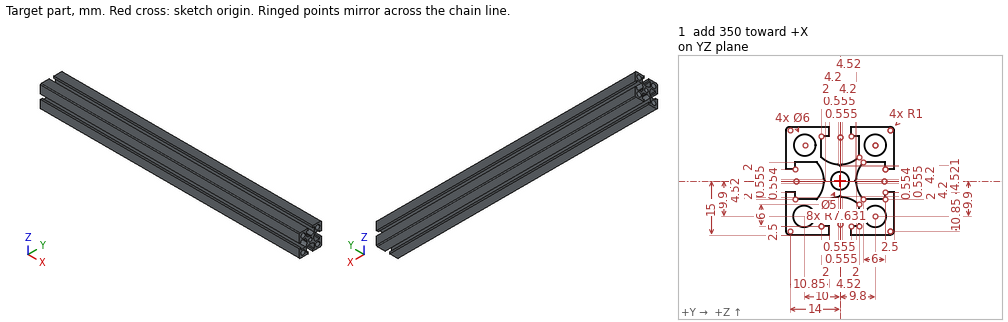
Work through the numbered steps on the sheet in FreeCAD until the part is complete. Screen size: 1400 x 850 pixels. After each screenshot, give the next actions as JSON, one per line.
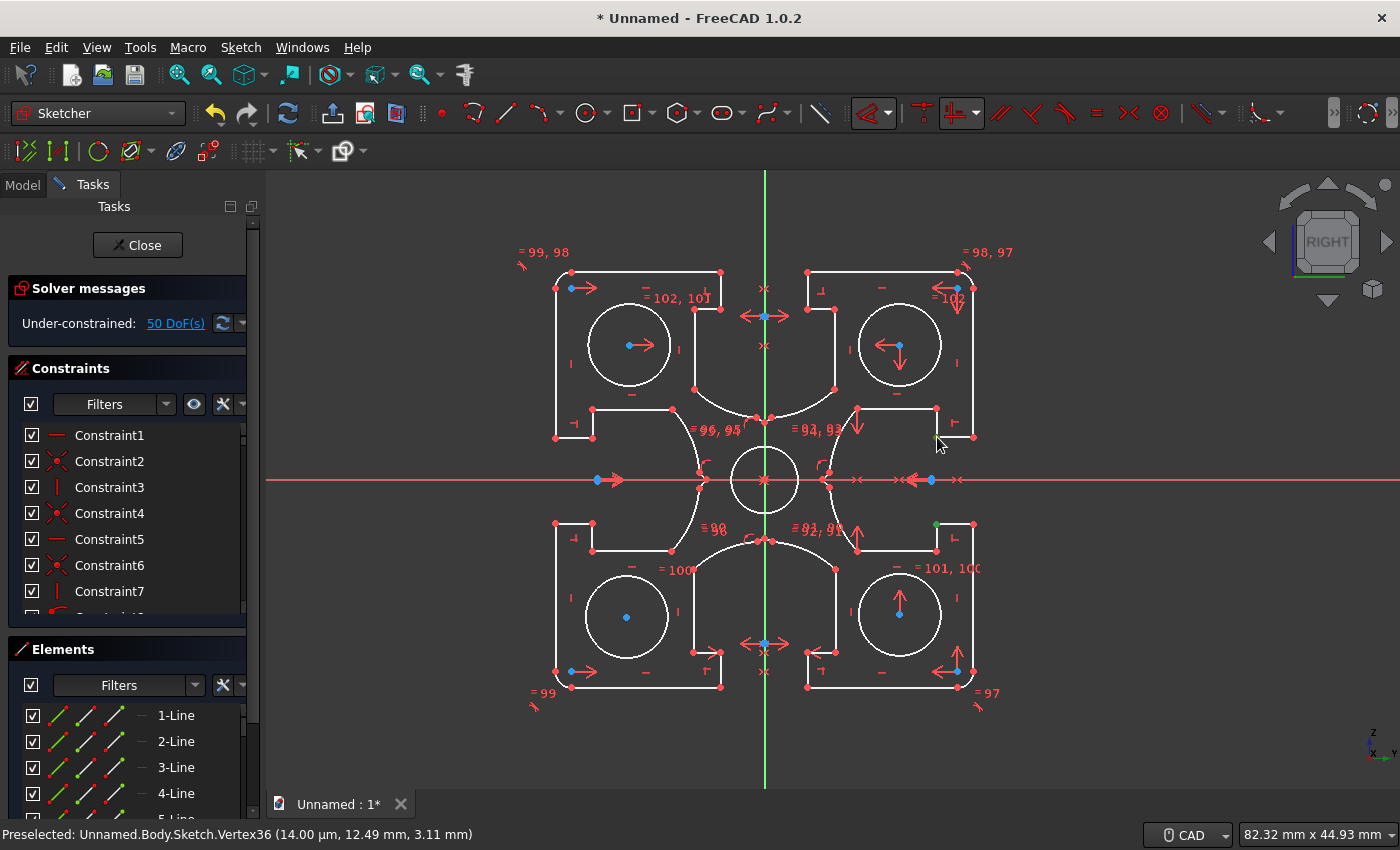
{"action": "left_click", "coordinate": [361, 480]}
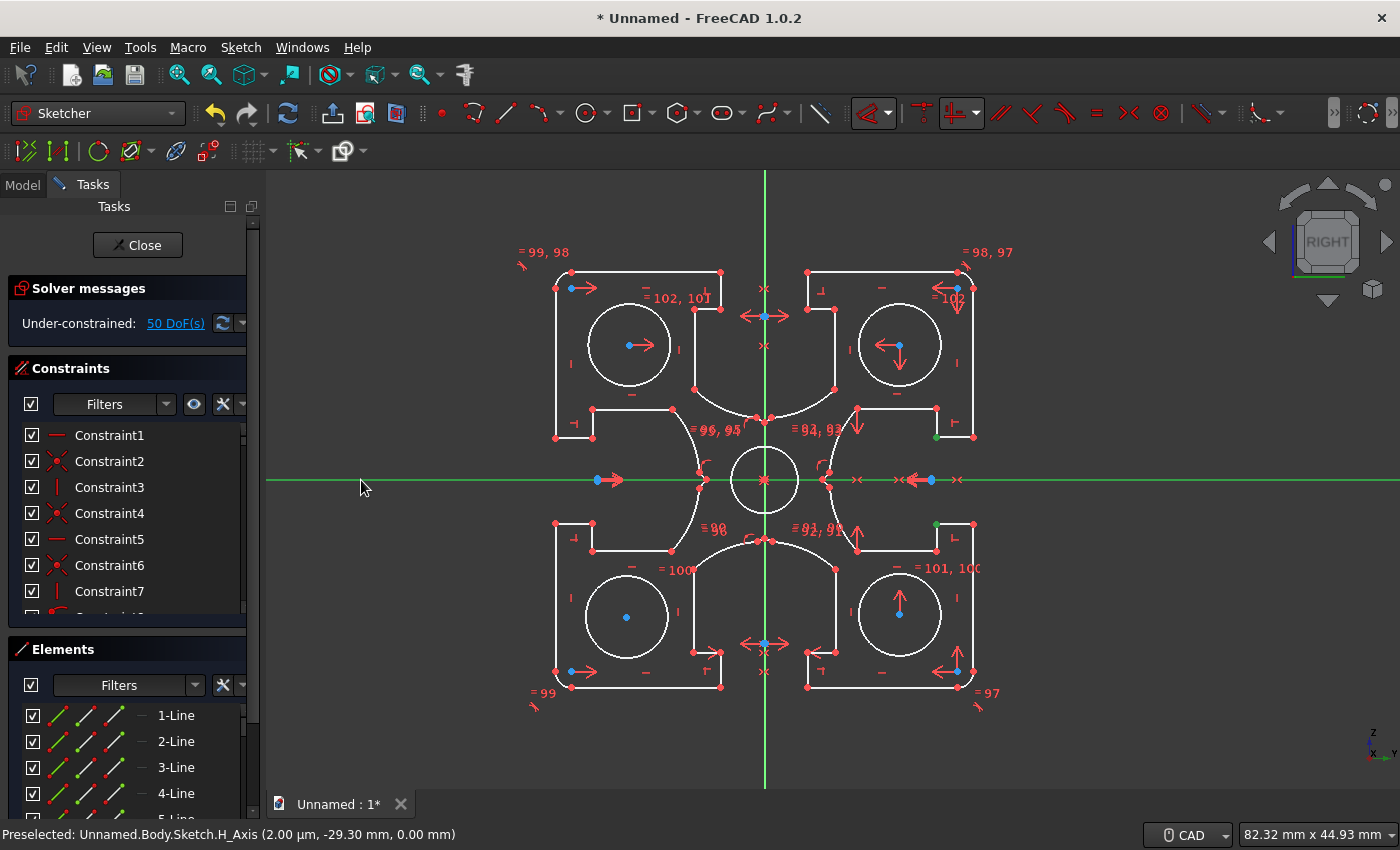
{"action": "left_click", "coordinate": [1130, 114]}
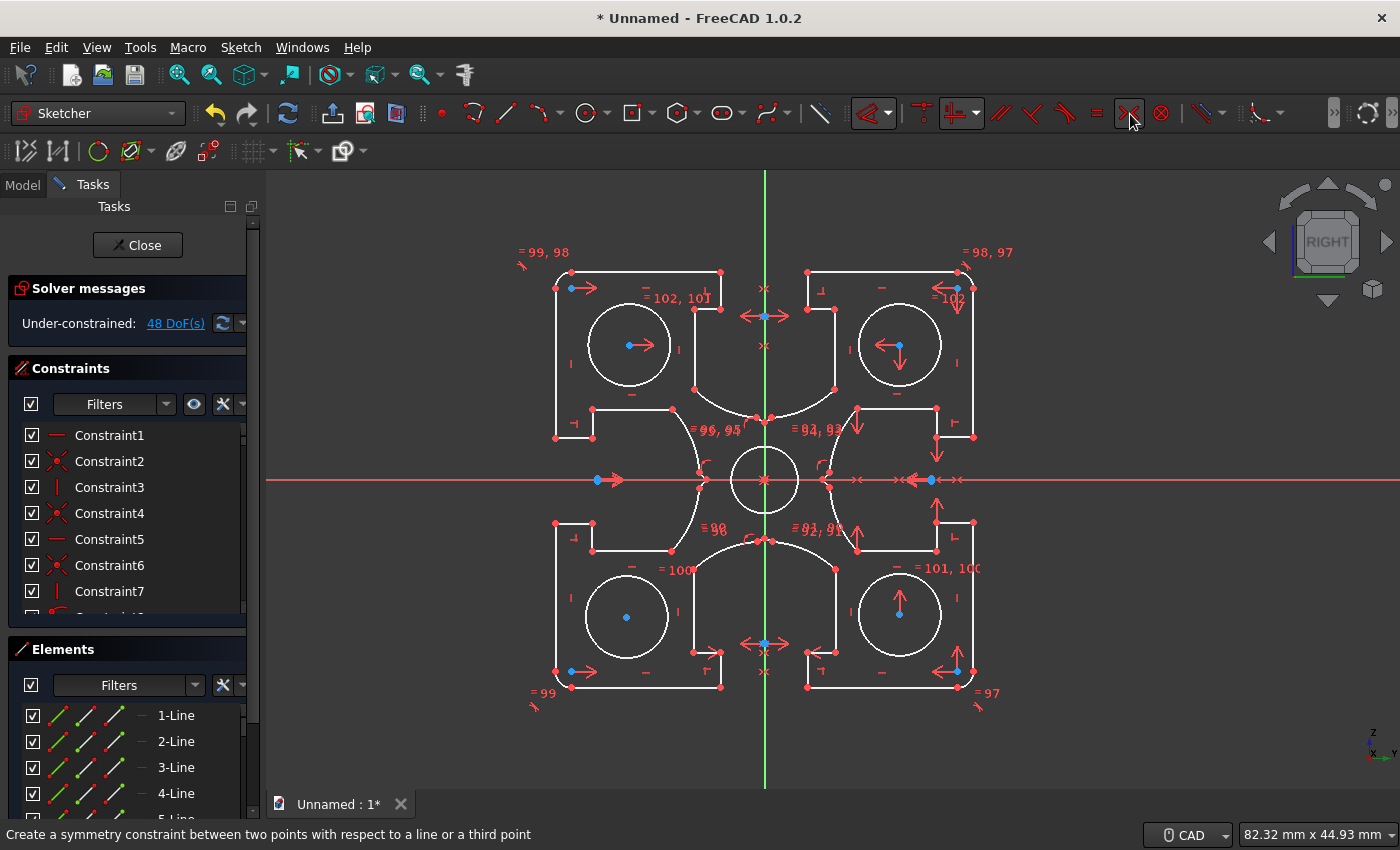
{"action": "left_click", "coordinate": [808, 653]}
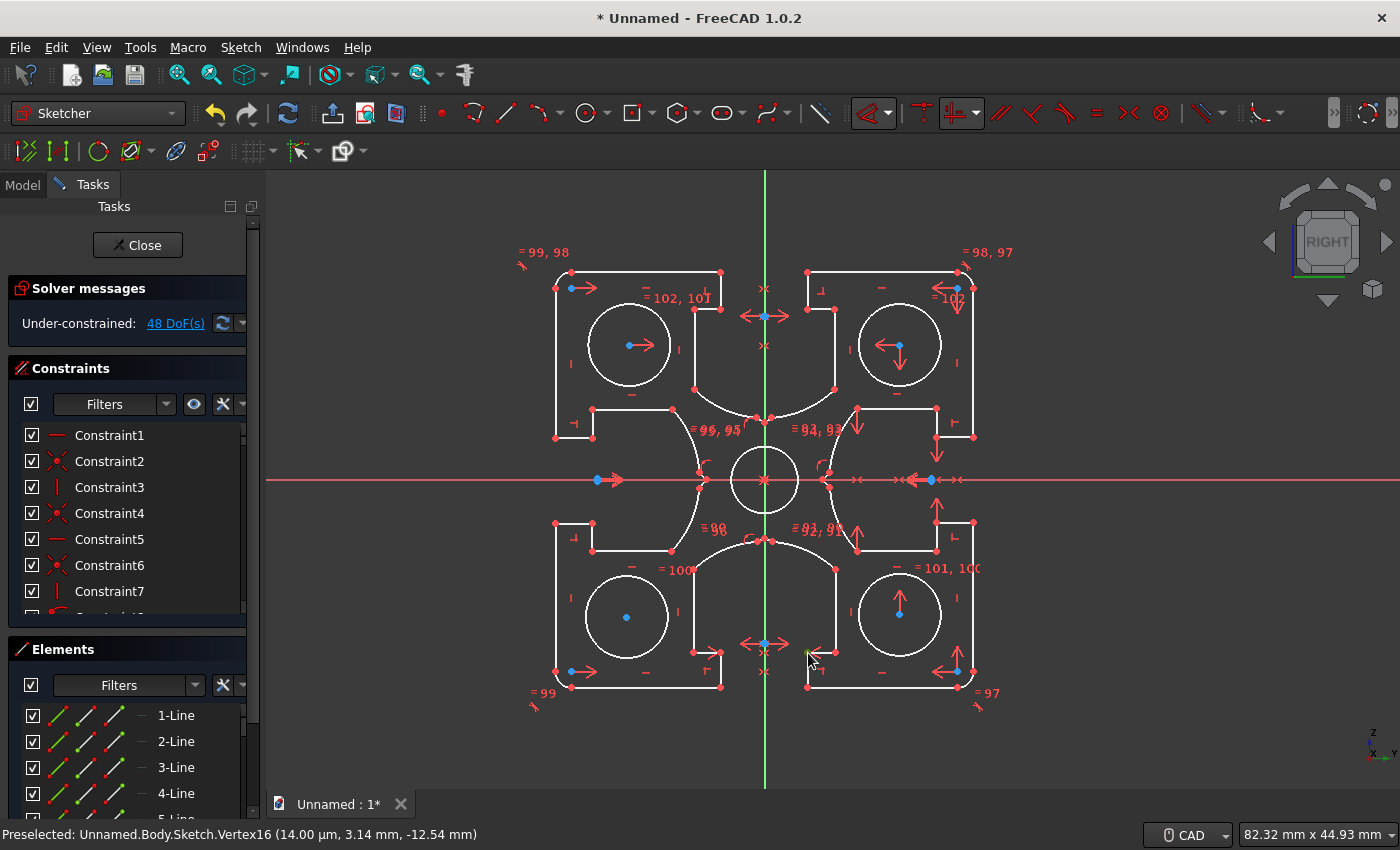
{"action": "left_click", "coordinate": [808, 309]}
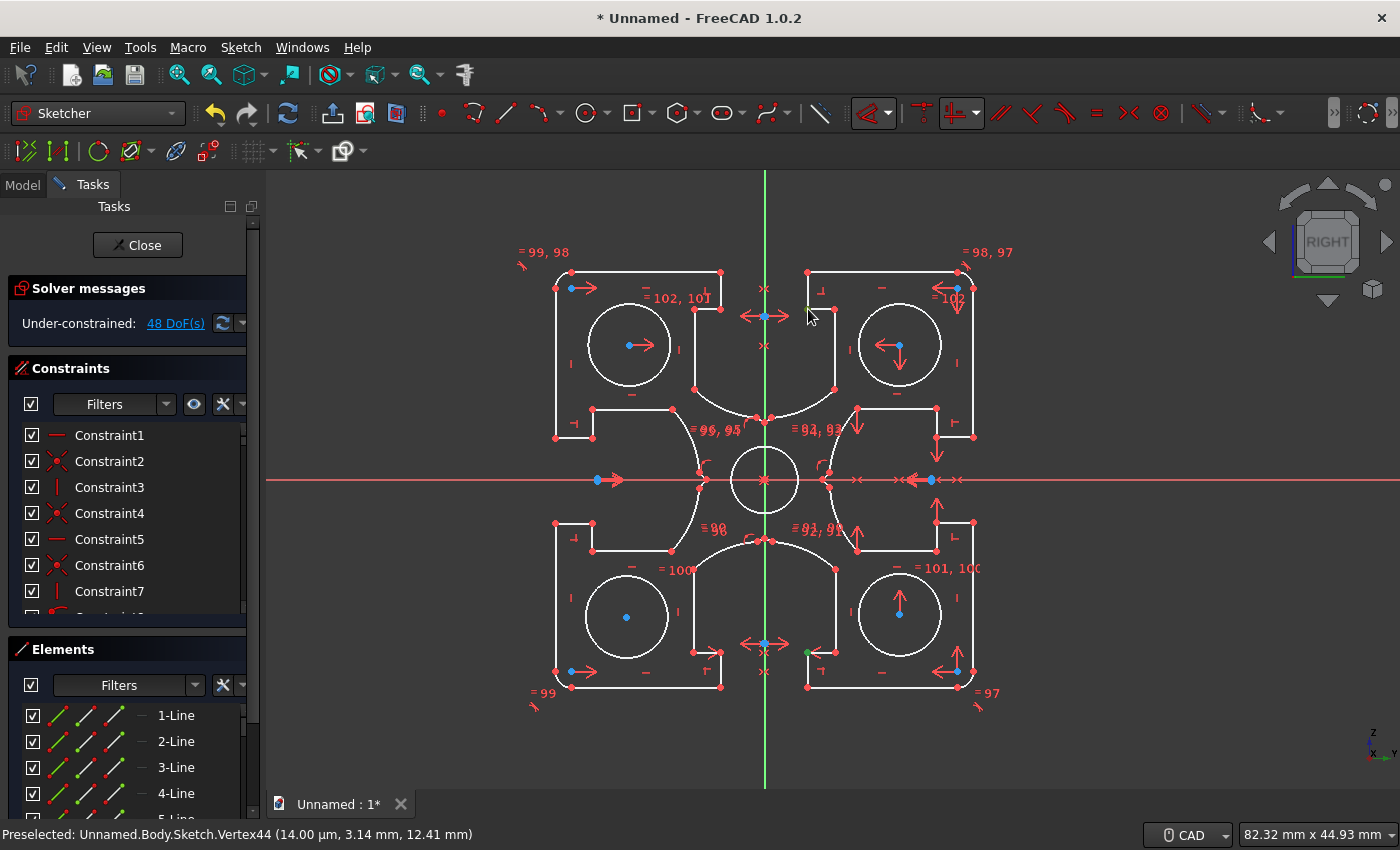
{"action": "left_click", "coordinate": [361, 480]}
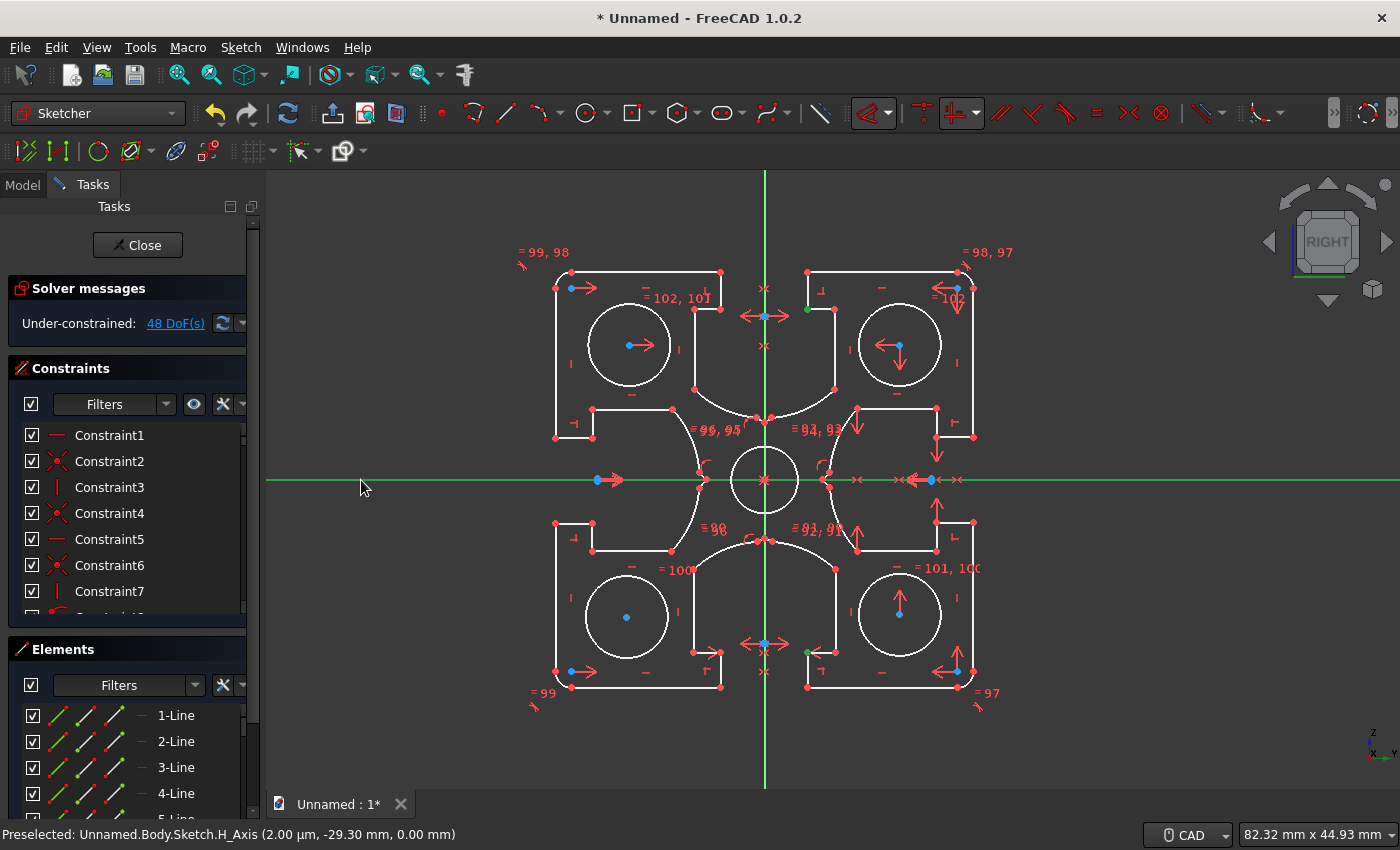
{"action": "left_click", "coordinate": [1130, 114]}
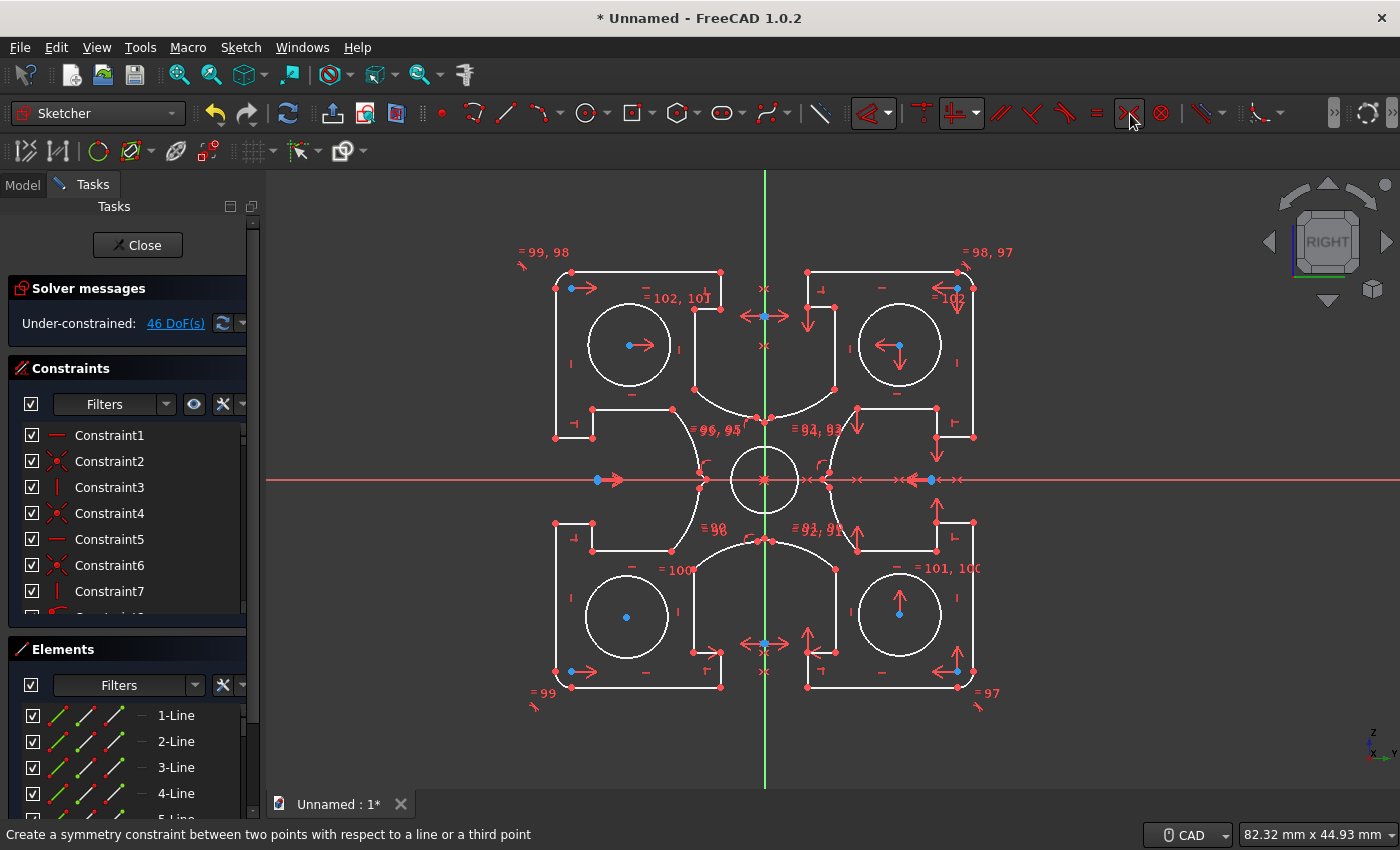
{"action": "left_click", "coordinate": [836, 570]}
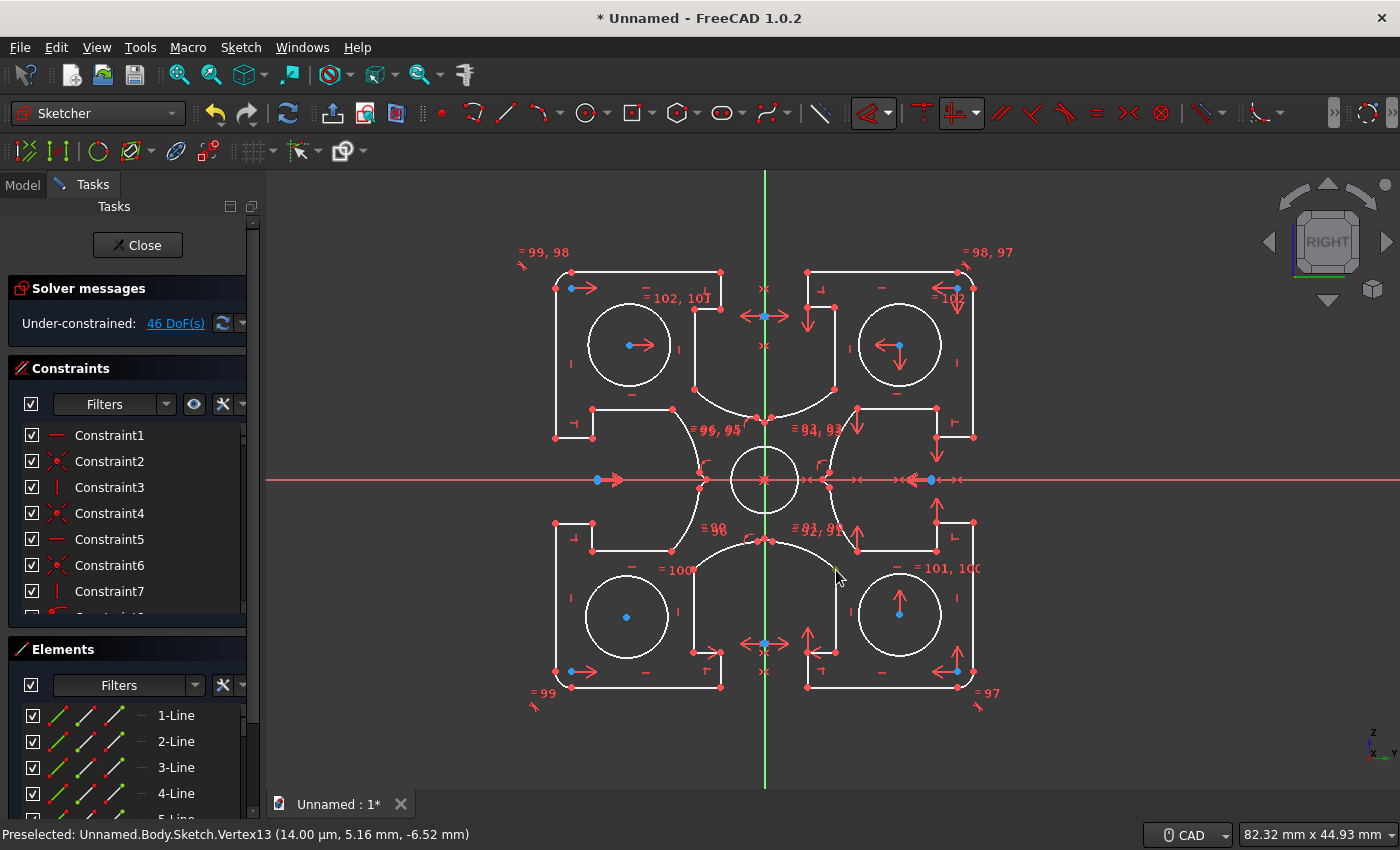
{"action": "left_click", "coordinate": [835, 390]}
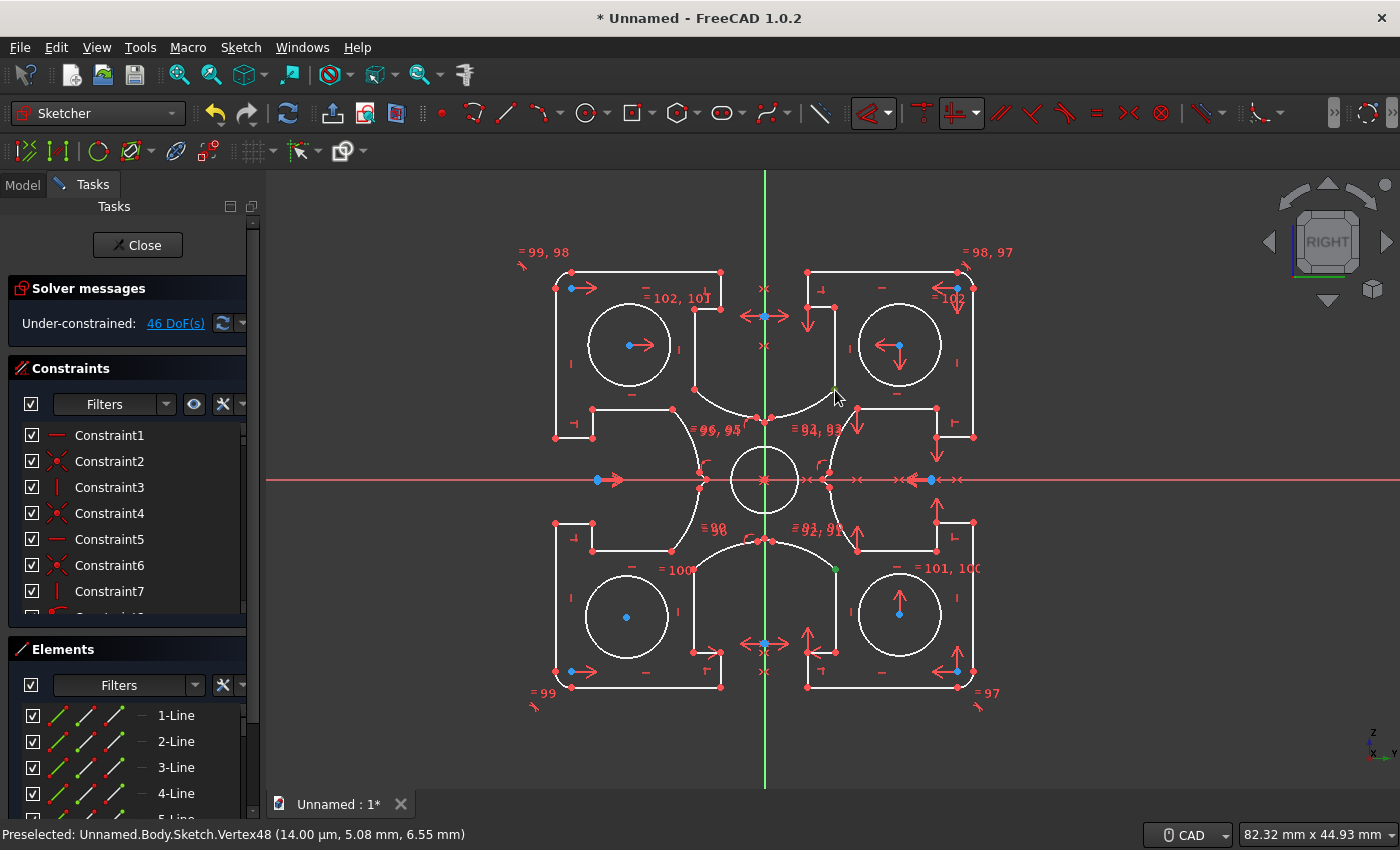
{"action": "left_click", "coordinate": [361, 480]}